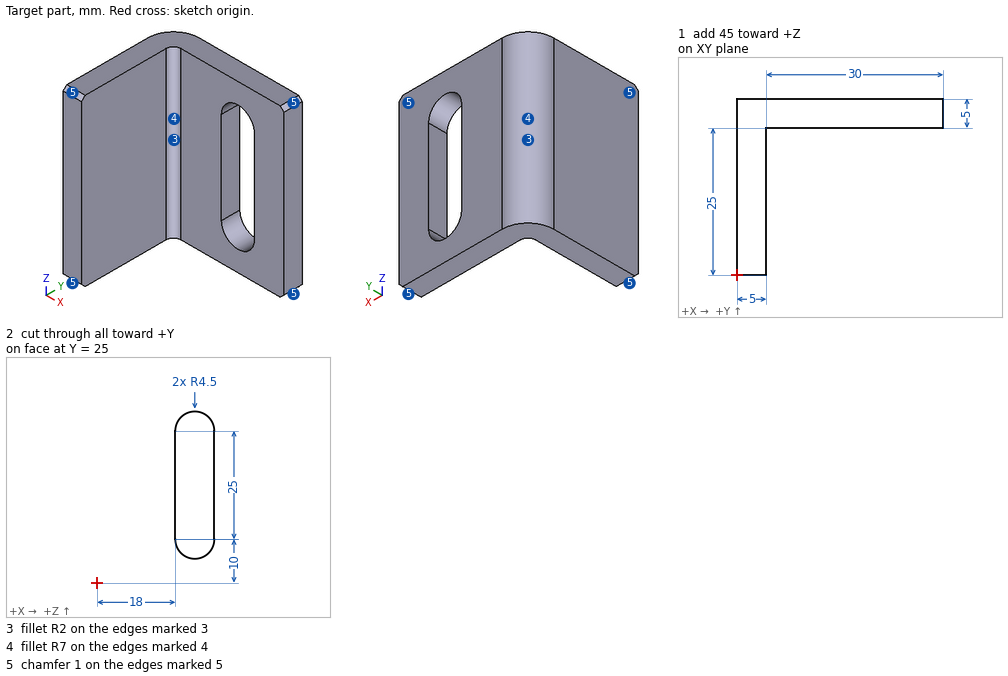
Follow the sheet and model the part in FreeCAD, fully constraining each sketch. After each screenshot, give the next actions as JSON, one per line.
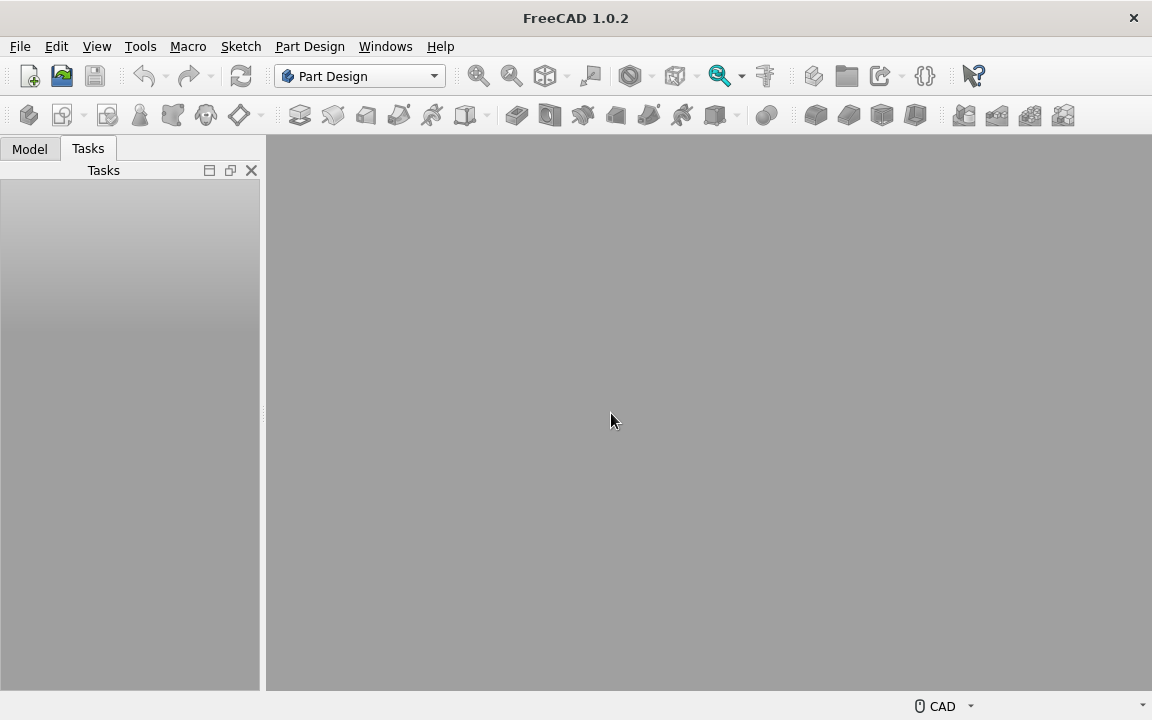
{"action": "key", "text": "ctrl+n"}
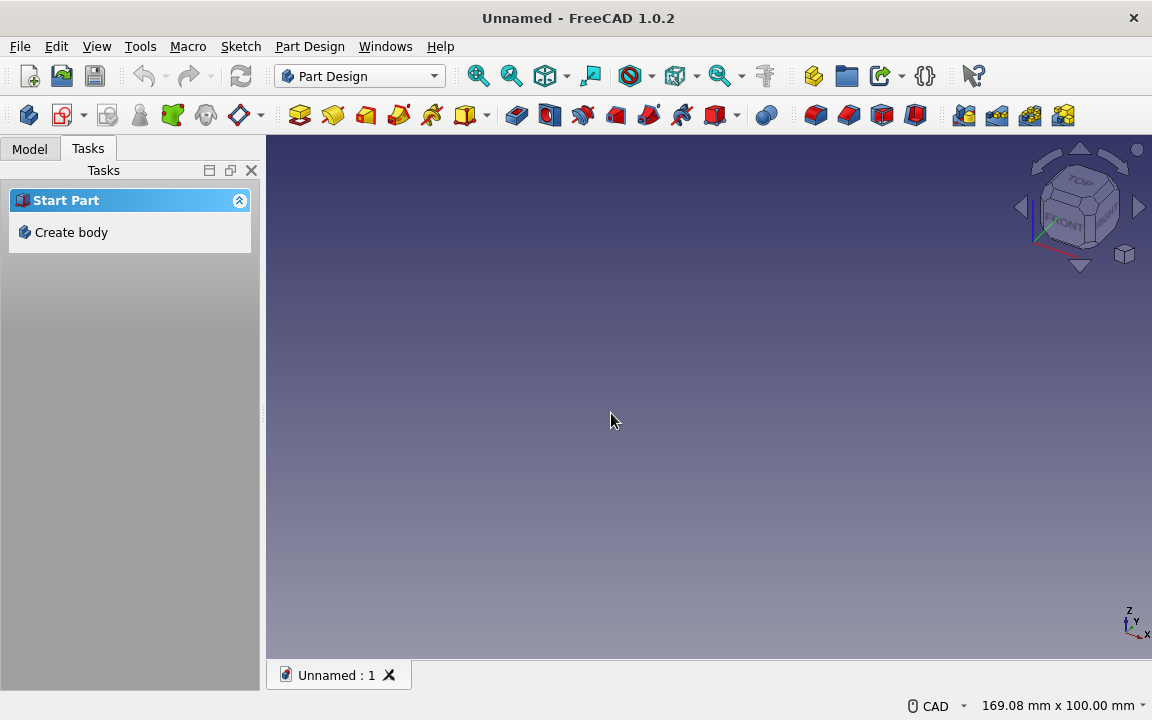
{"action": "left_click", "coordinate": [62, 116]}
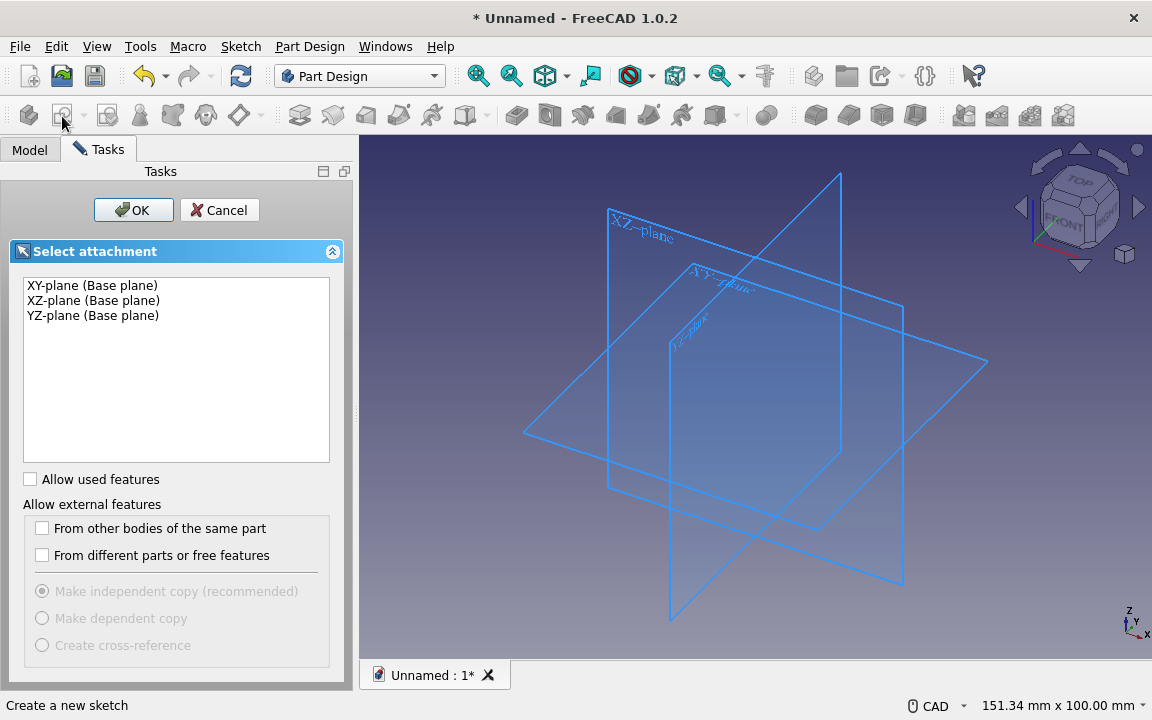
{"action": "left_click", "coordinate": [84, 286]}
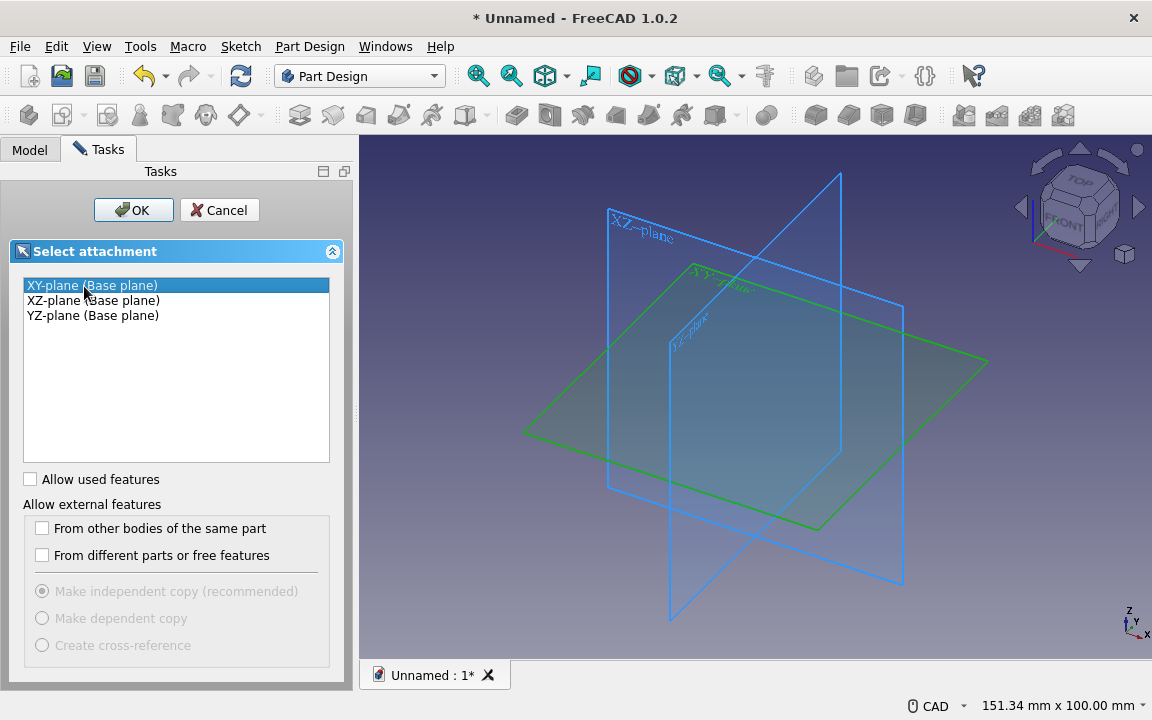
{"action": "left_click", "coordinate": [134, 210]}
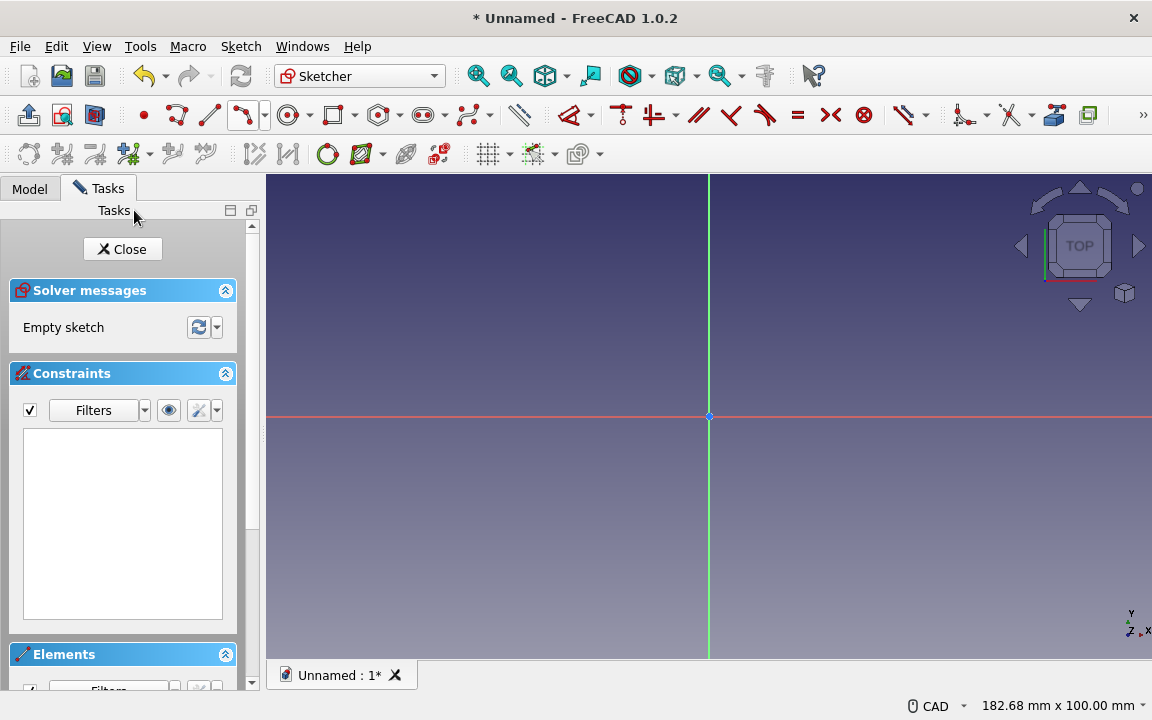
{"action": "scroll", "coordinate": [919, 284], "scroll_direction": "up", "scroll_amount": 4}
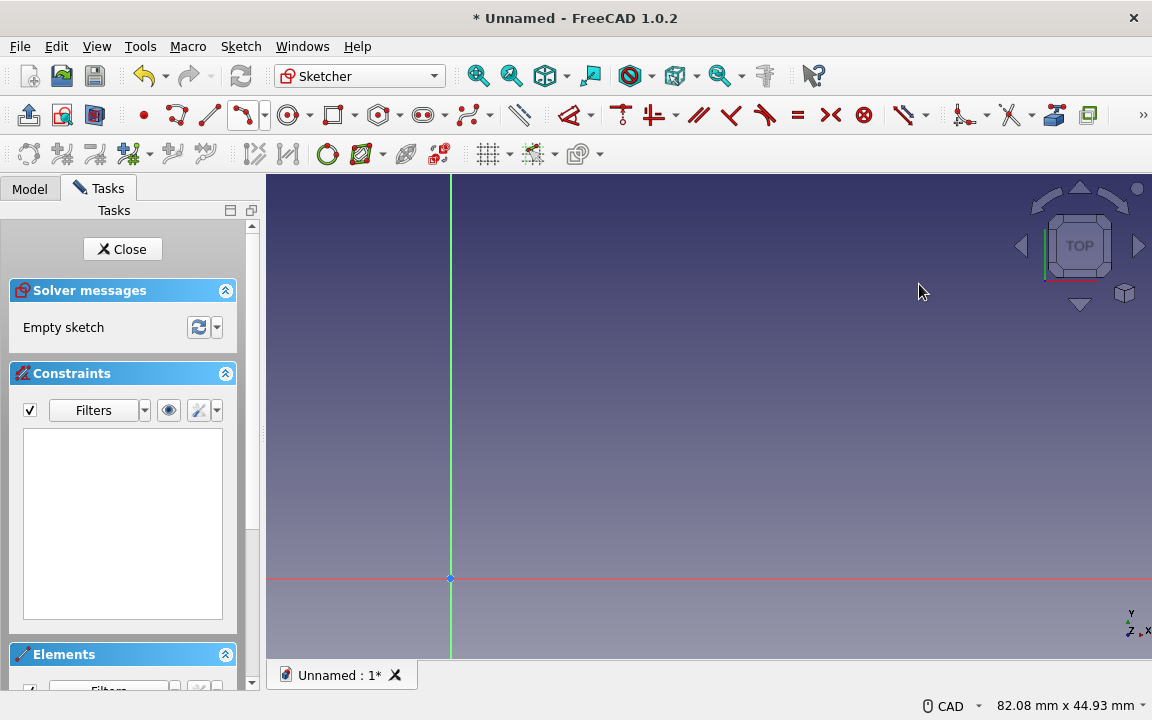
{"action": "key", "text": "g m"}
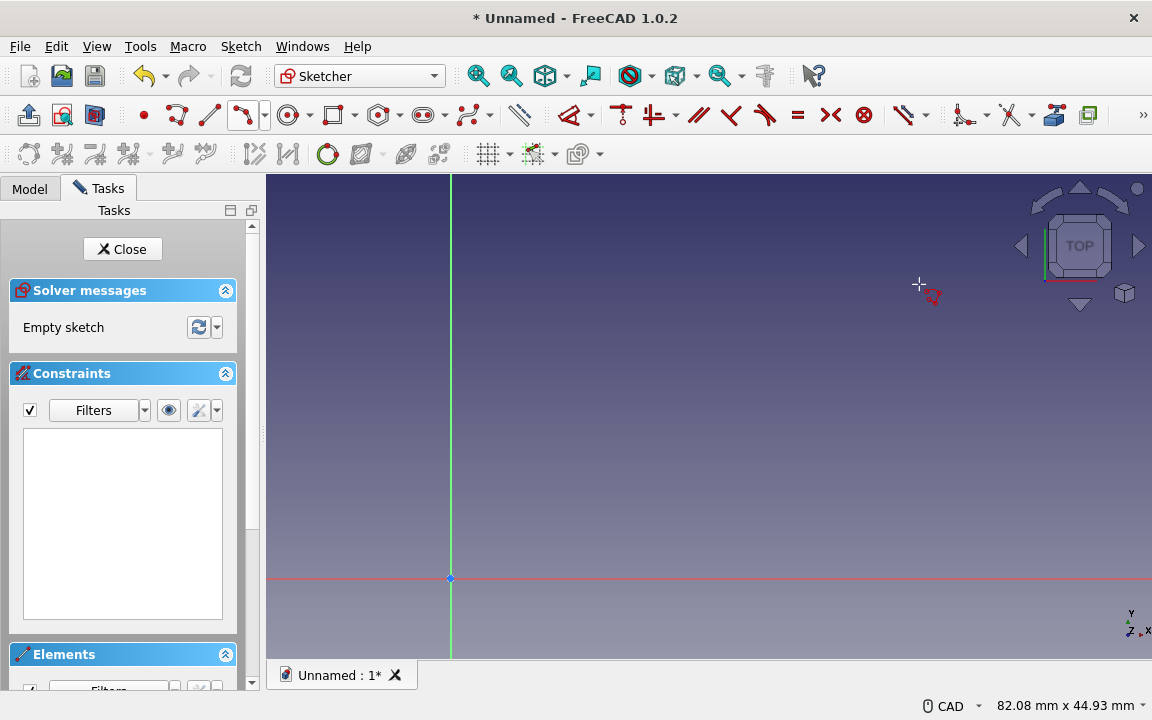
{"action": "left_click", "coordinate": [451, 579]}
{"action": "left_click", "coordinate": [505, 570]}
{"action": "left_click", "coordinate": [505, 309]}
{"action": "left_click", "coordinate": [829, 309]}
{"action": "left_click", "coordinate": [829, 255]}
{"action": "left_click", "coordinate": [460, 255]}
{"action": "left_click", "coordinate": [451, 579]}
{"action": "key", "text": "Escape"}
{"action": "key", "text": "Escape"}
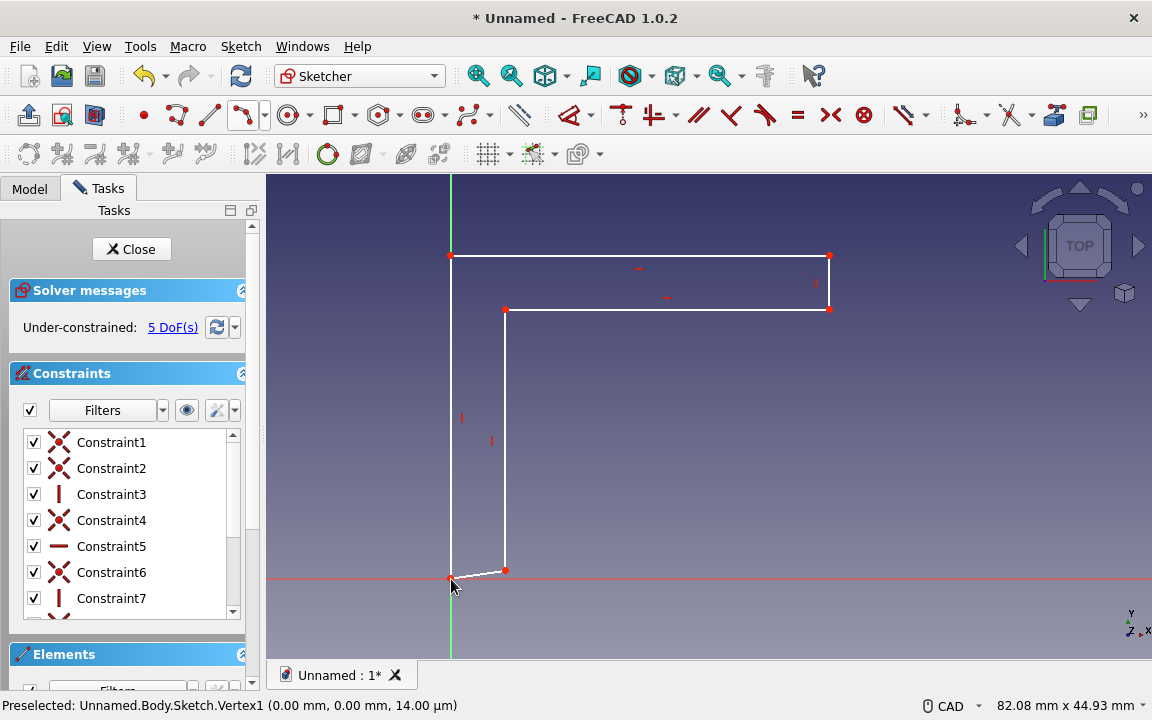
{"action": "left_click", "coordinate": [467, 576]}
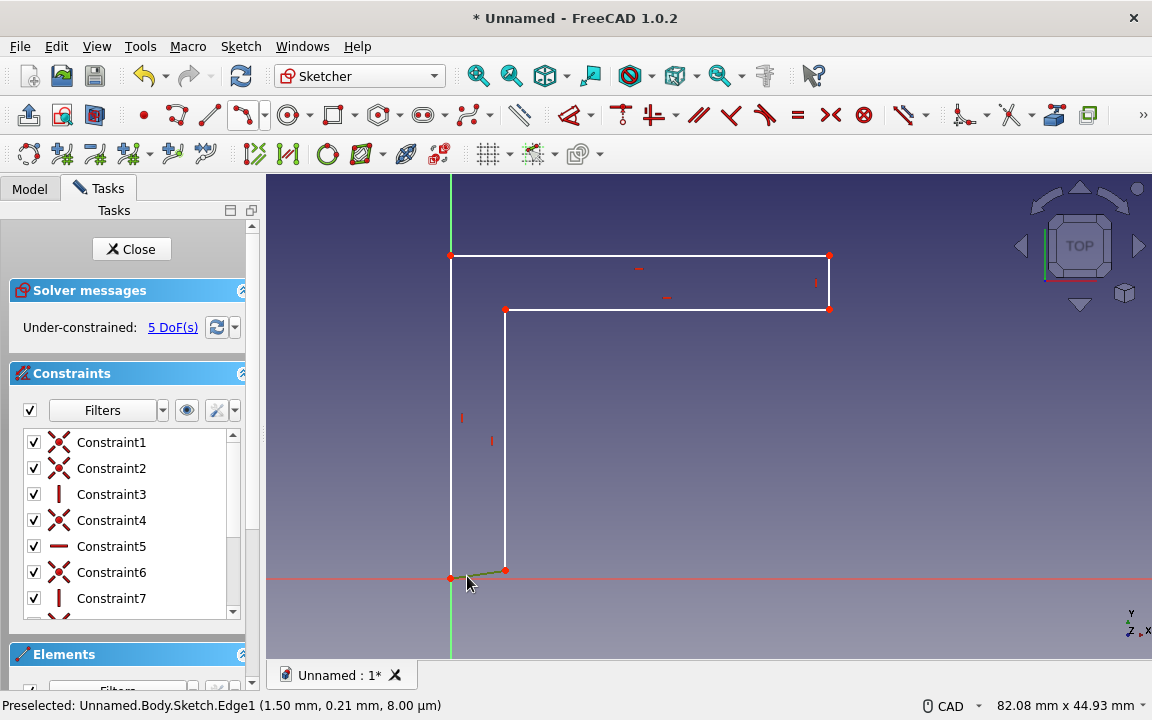
{"action": "key", "text": "h"}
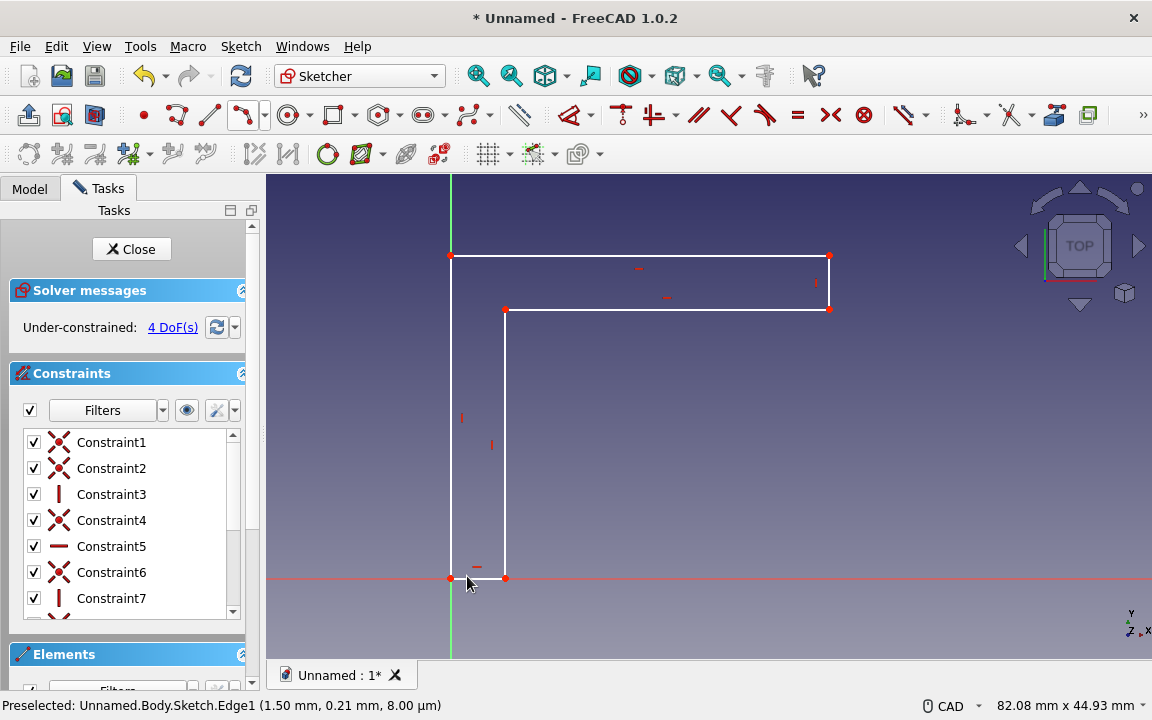
{"action": "key", "text": "d"}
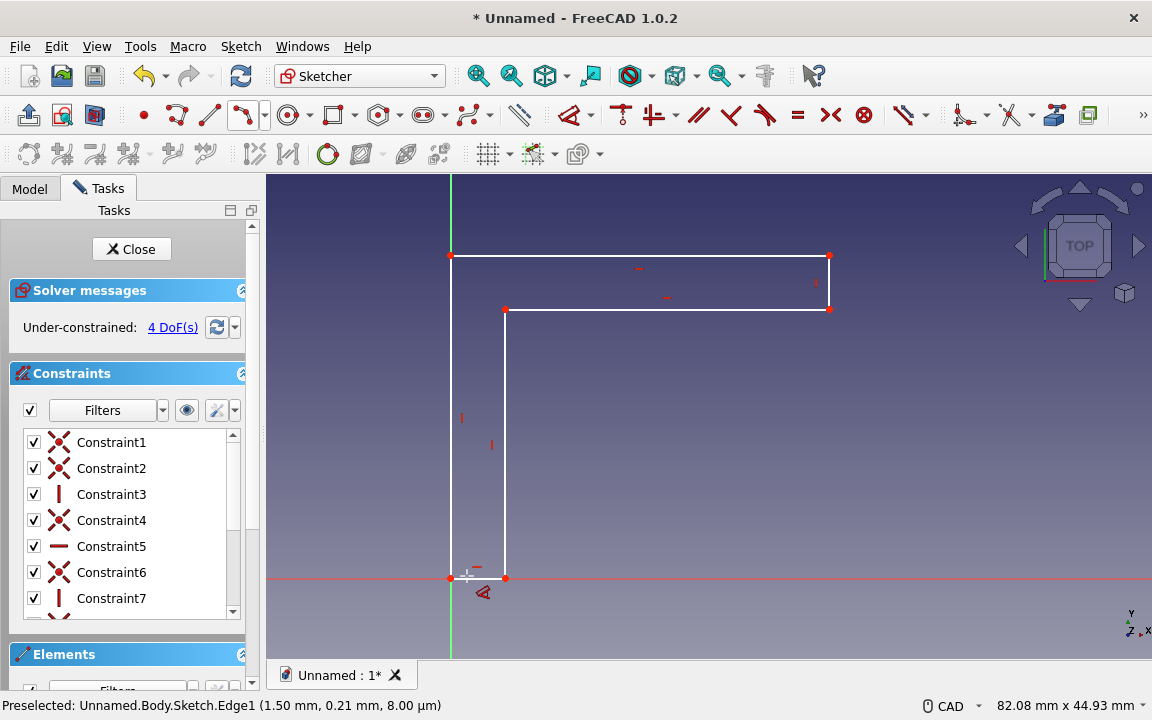
{"action": "left_click", "coordinate": [467, 579]}
{"action": "left_click", "coordinate": [478, 613]}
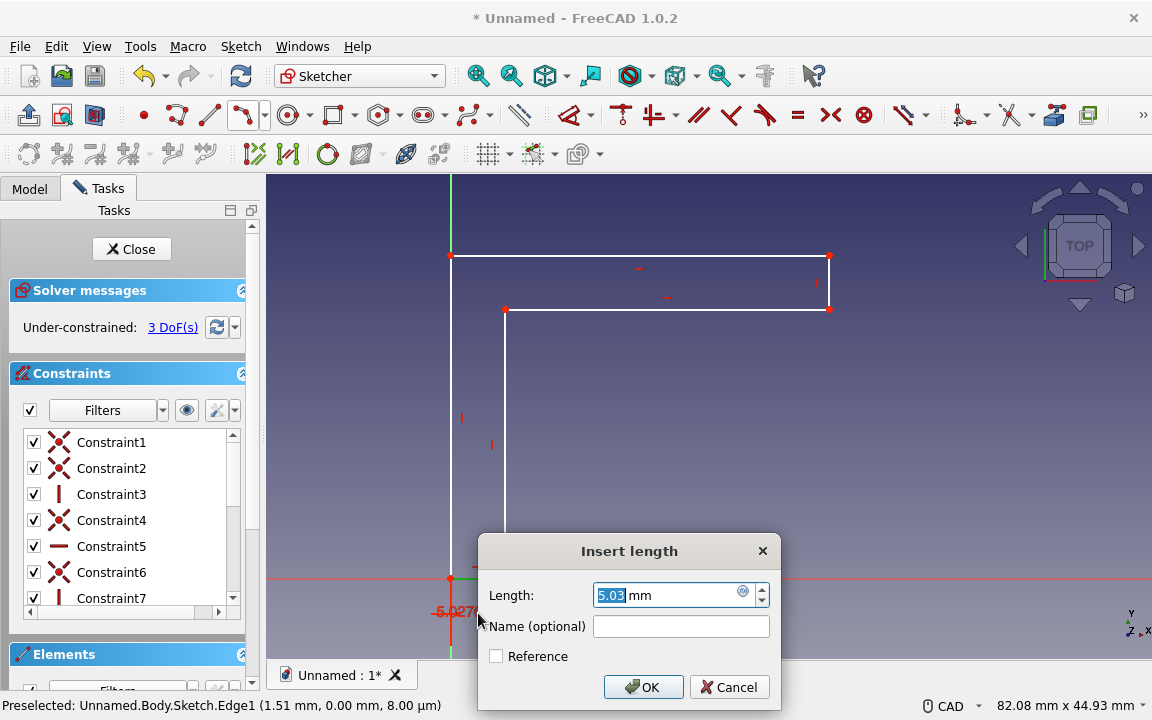
{"action": "type", "text": "5"}
{"action": "key", "text": "Return"}